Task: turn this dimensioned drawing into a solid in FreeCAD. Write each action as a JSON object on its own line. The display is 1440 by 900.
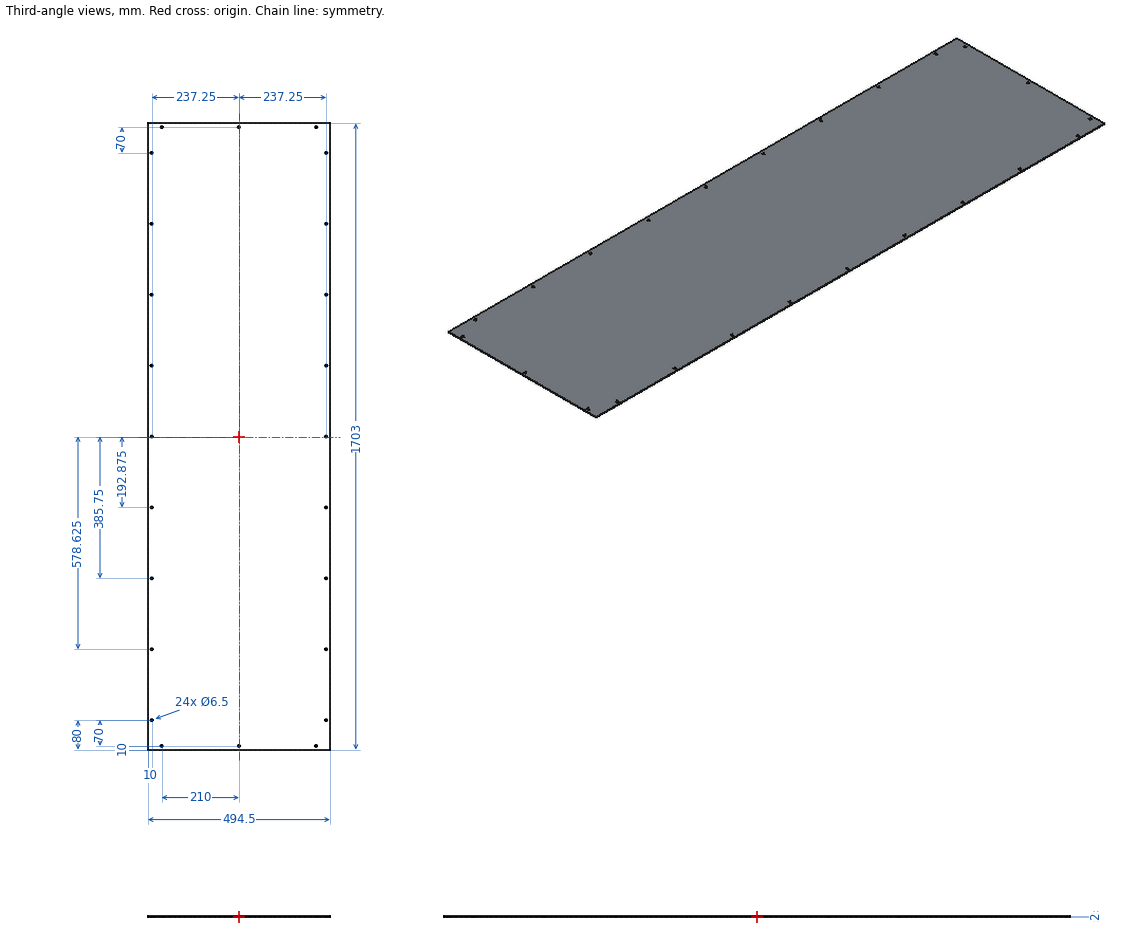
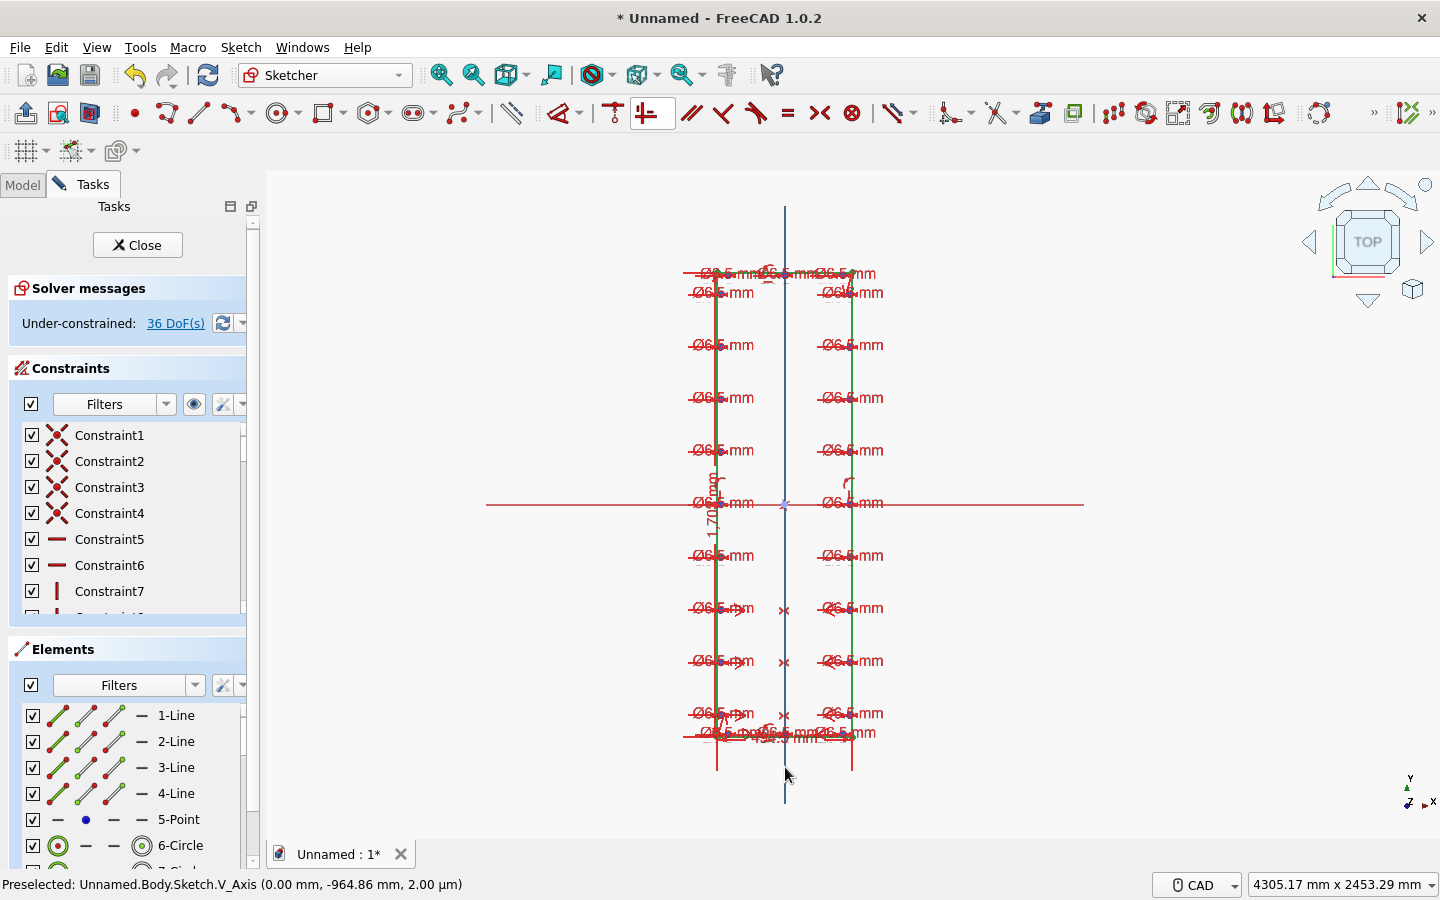
{"action": "left_click", "coordinate": [820, 114]}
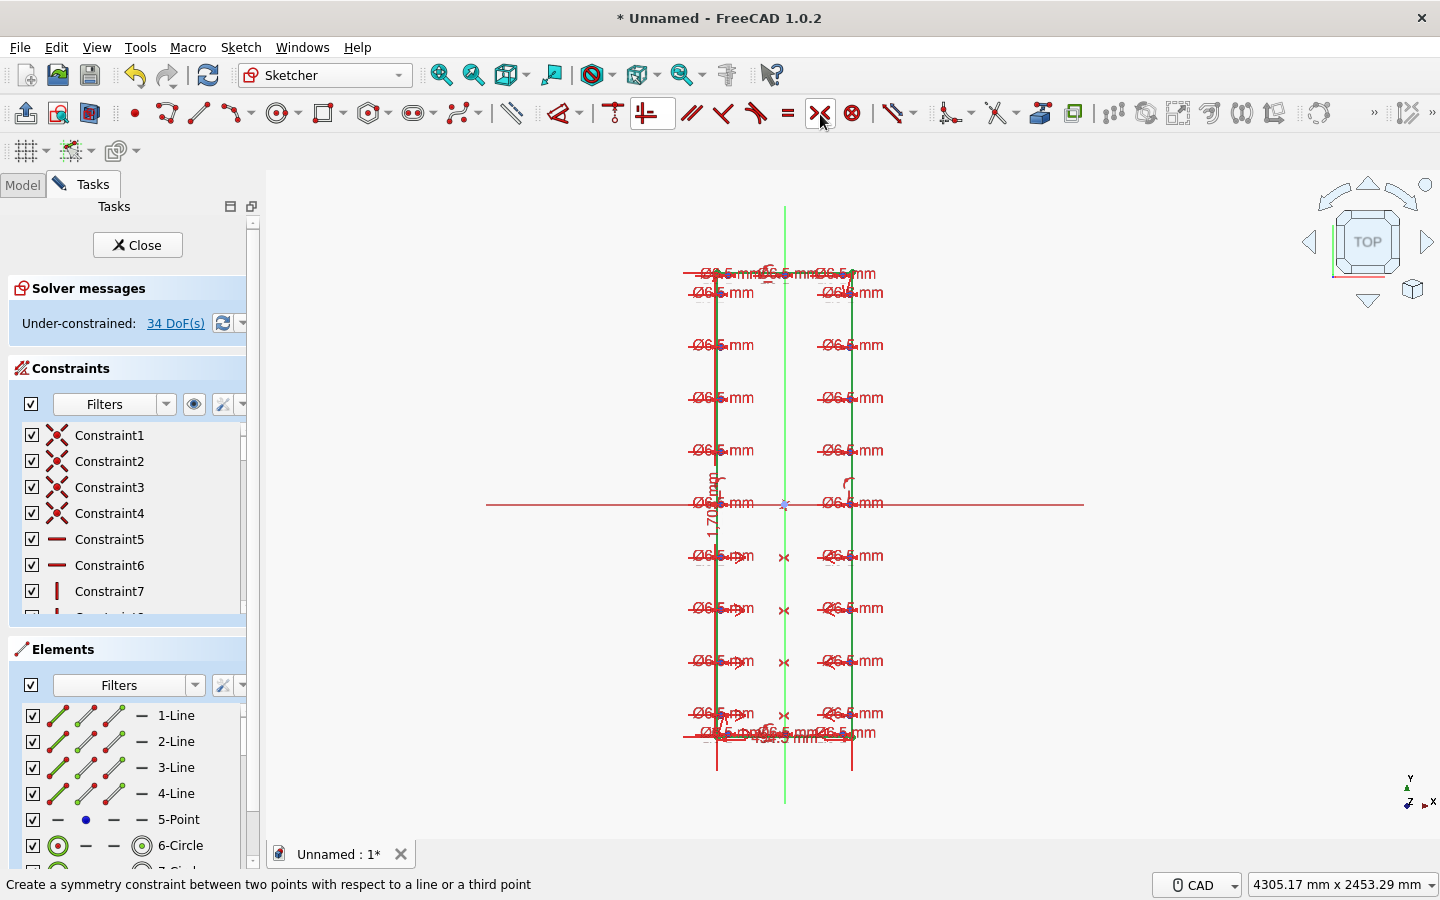
{"action": "left_click", "coordinate": [720, 558]}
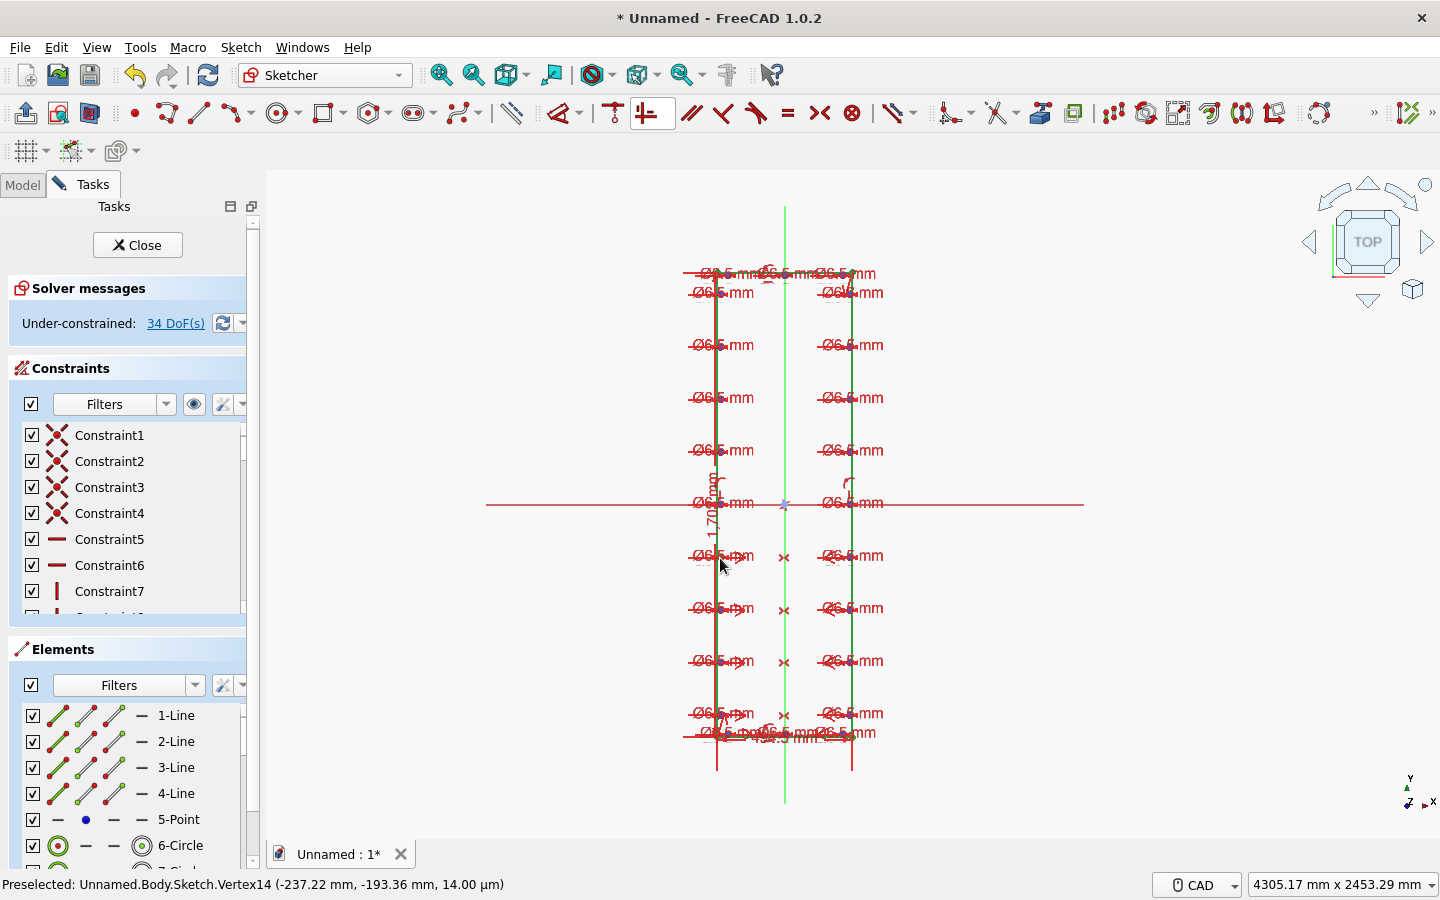
{"action": "left_click", "coordinate": [720, 452]}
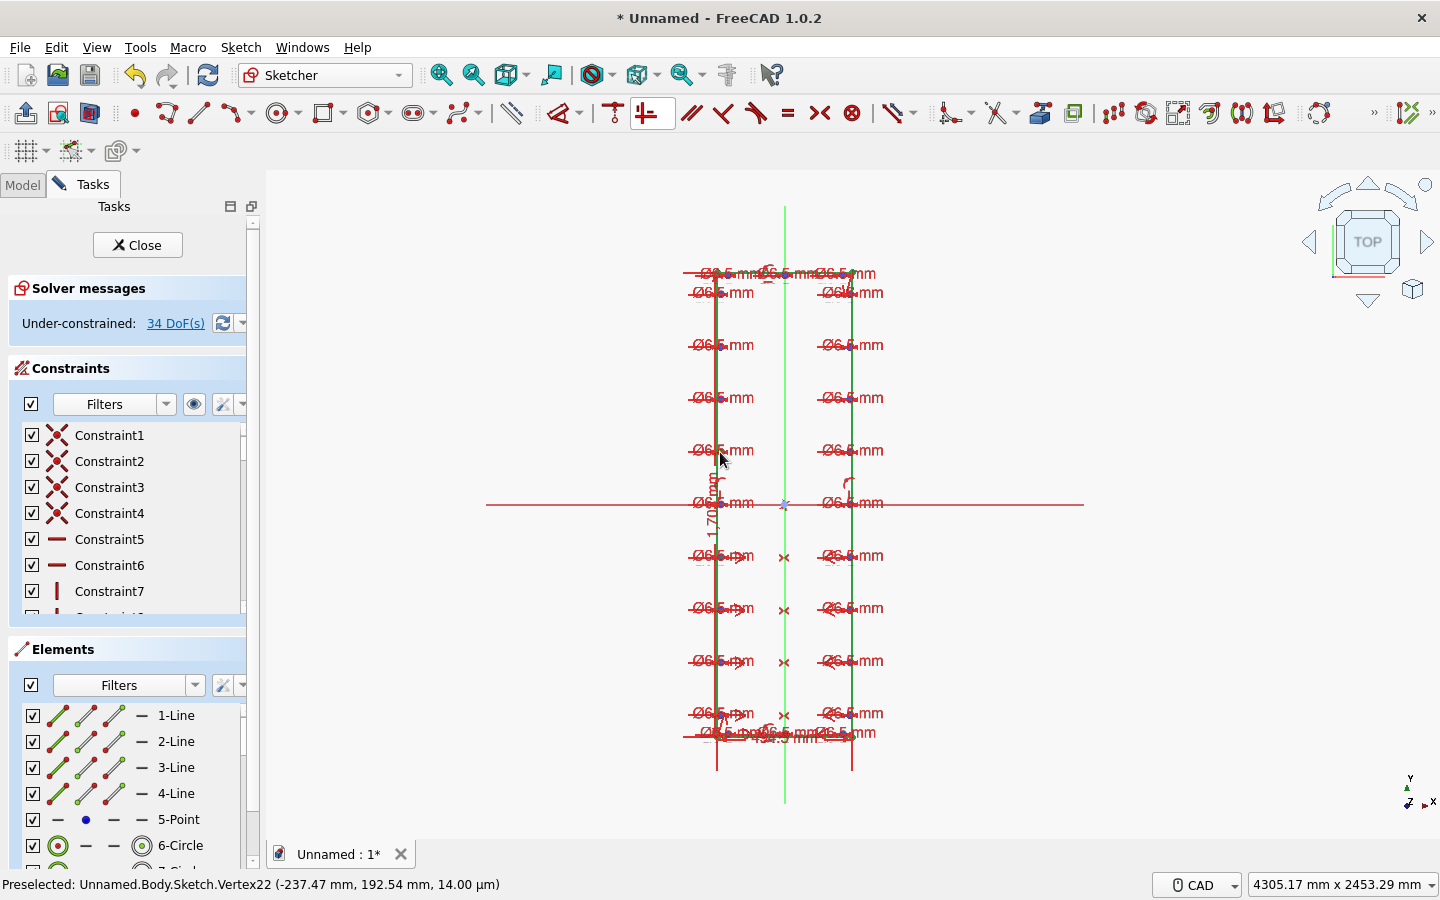
{"action": "left_click", "coordinate": [504, 505]}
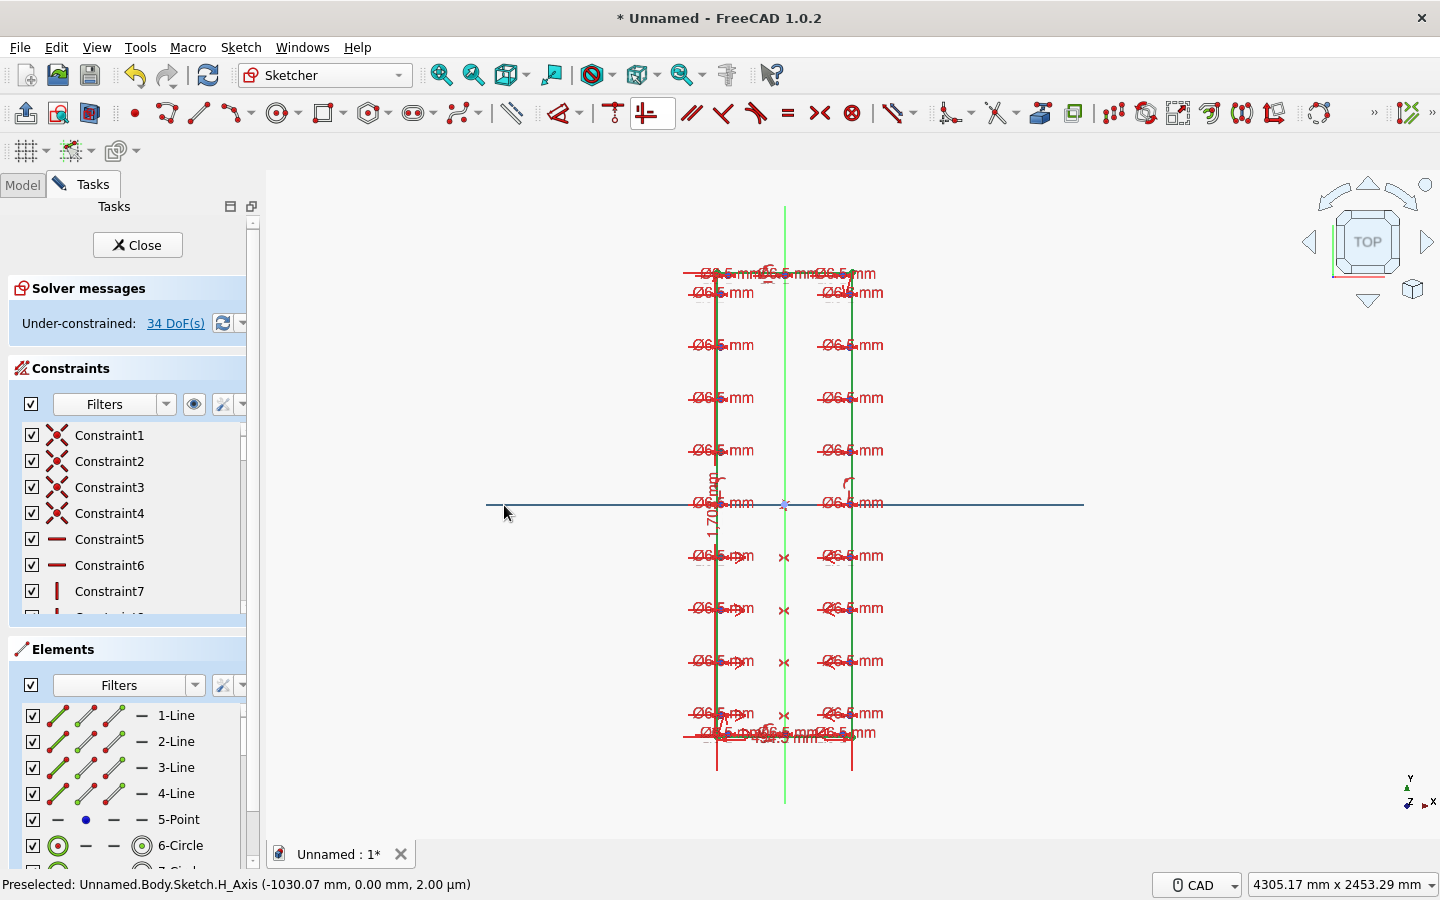
{"action": "left_click", "coordinate": [820, 114]}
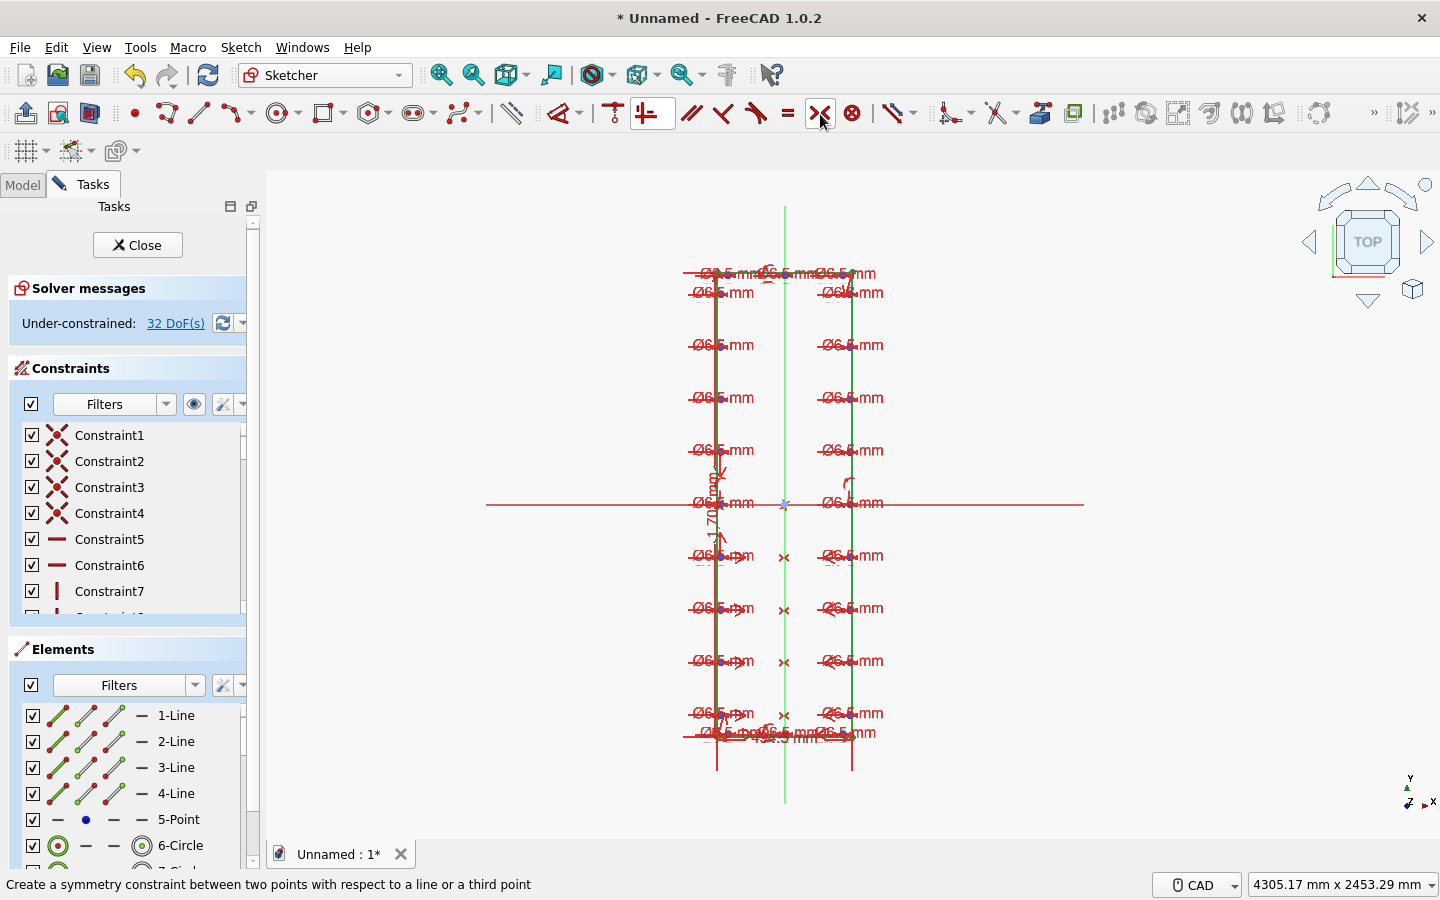
{"action": "left_click", "coordinate": [720, 610]}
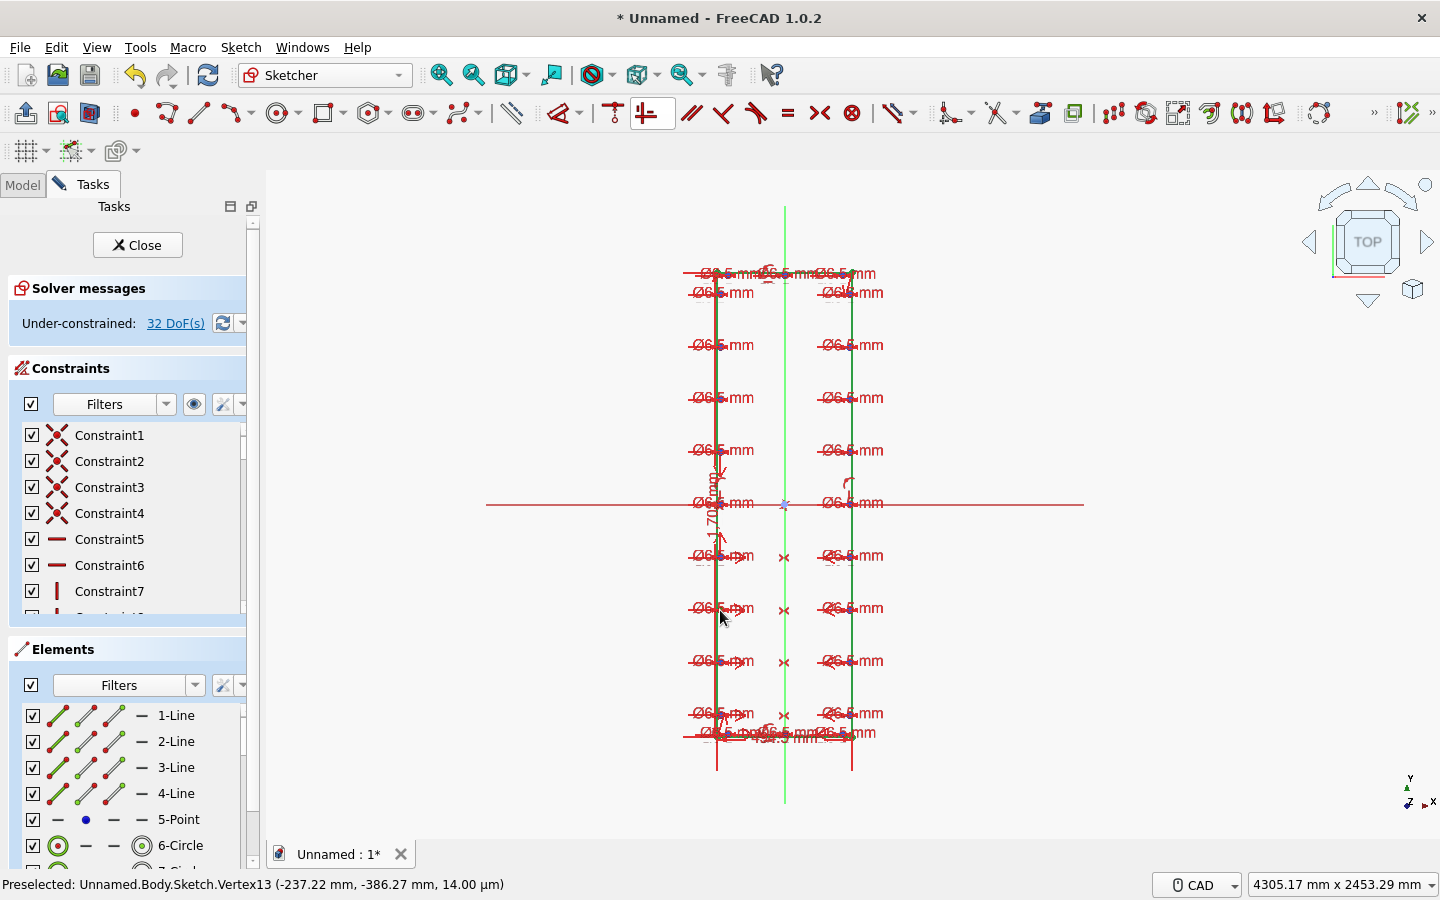
{"action": "left_click", "coordinate": [720, 400]}